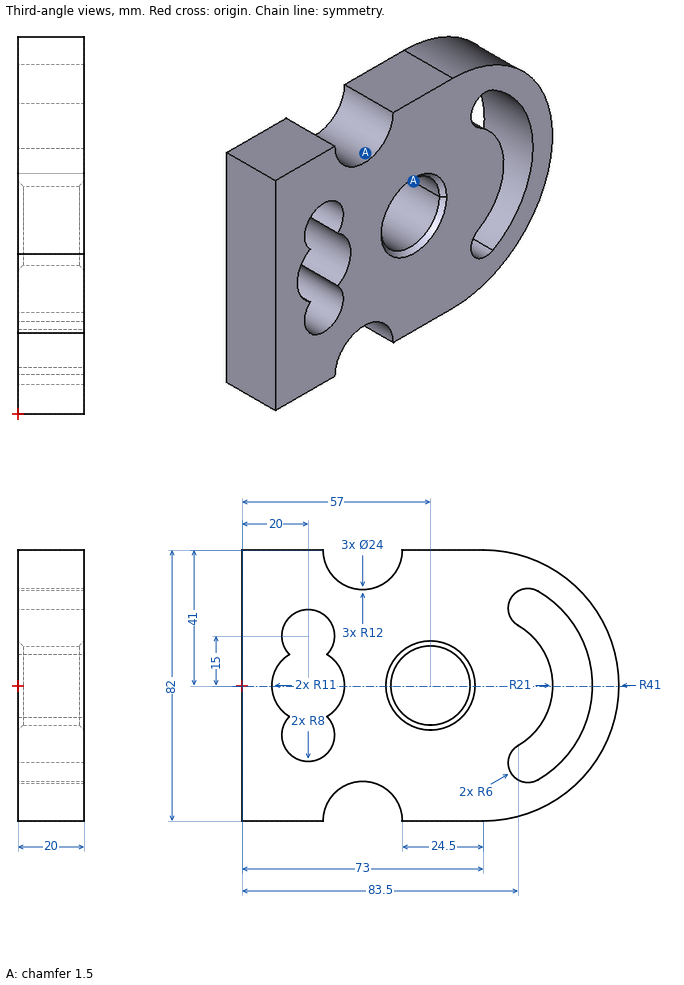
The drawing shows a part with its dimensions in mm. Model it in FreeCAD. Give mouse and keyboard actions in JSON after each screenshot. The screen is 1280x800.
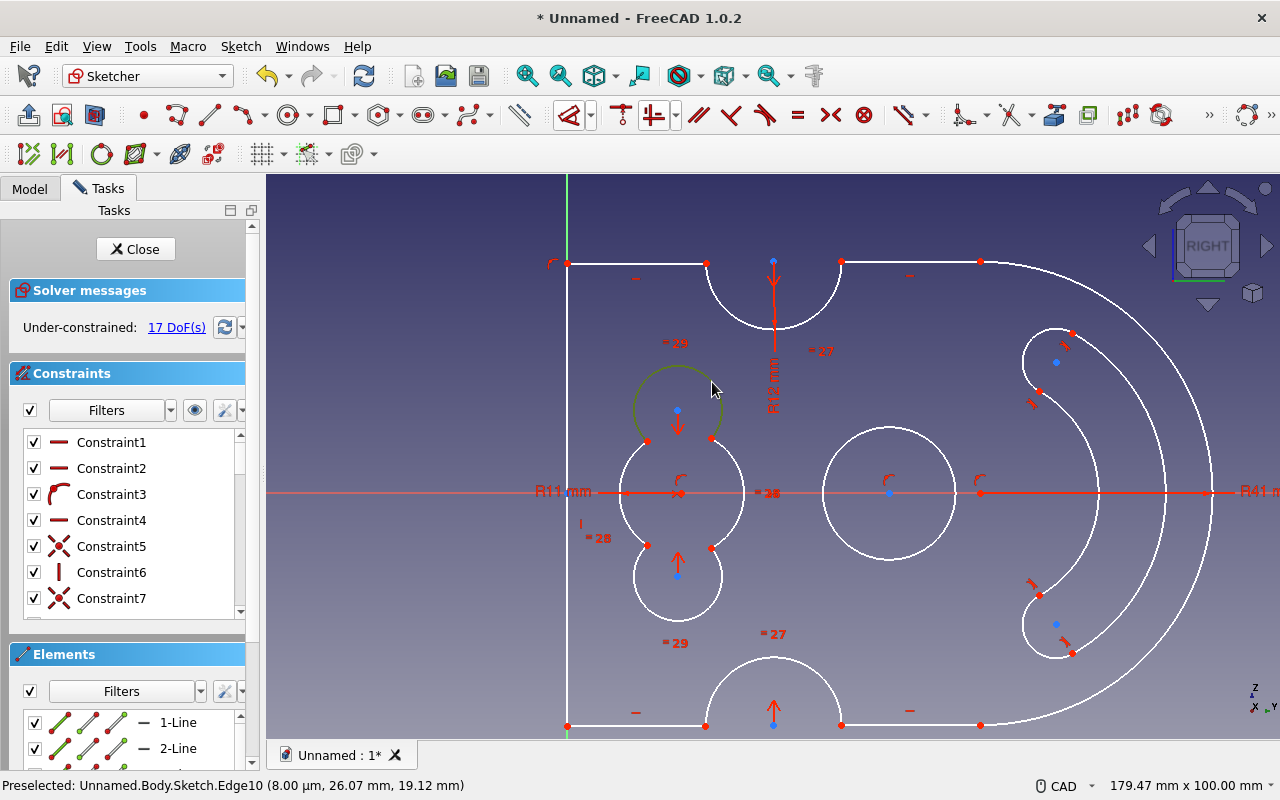
{"action": "key", "text": "k r"}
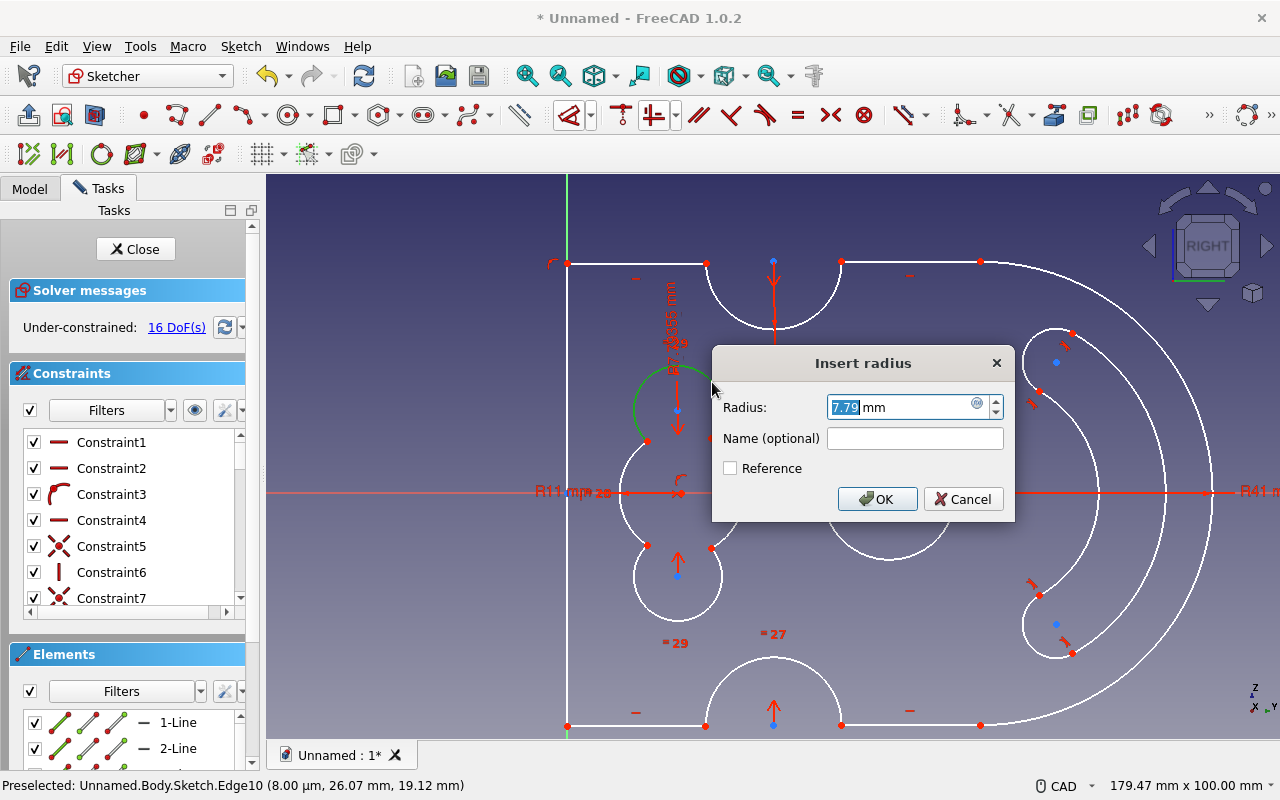
{"action": "type", "text": "8"}
{"action": "key", "text": "Return"}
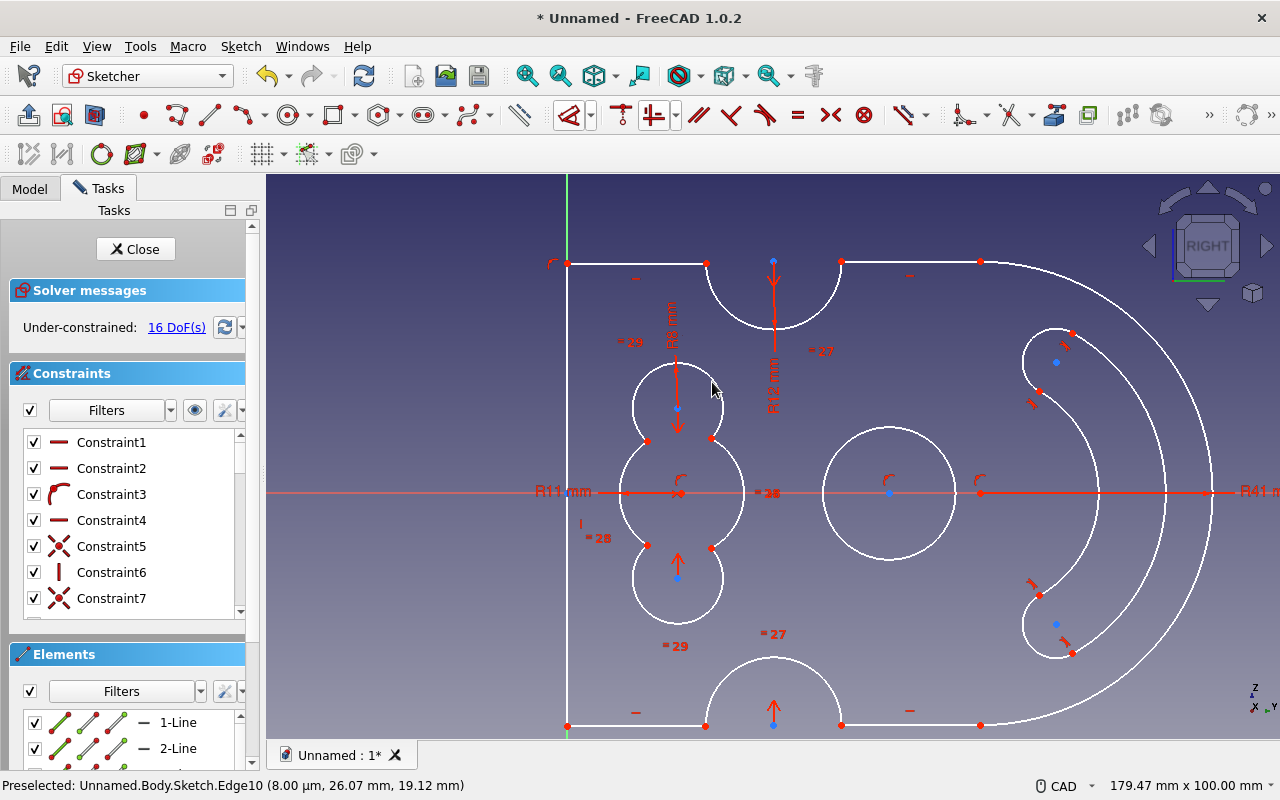
{"action": "left_click", "coordinate": [1088, 541]}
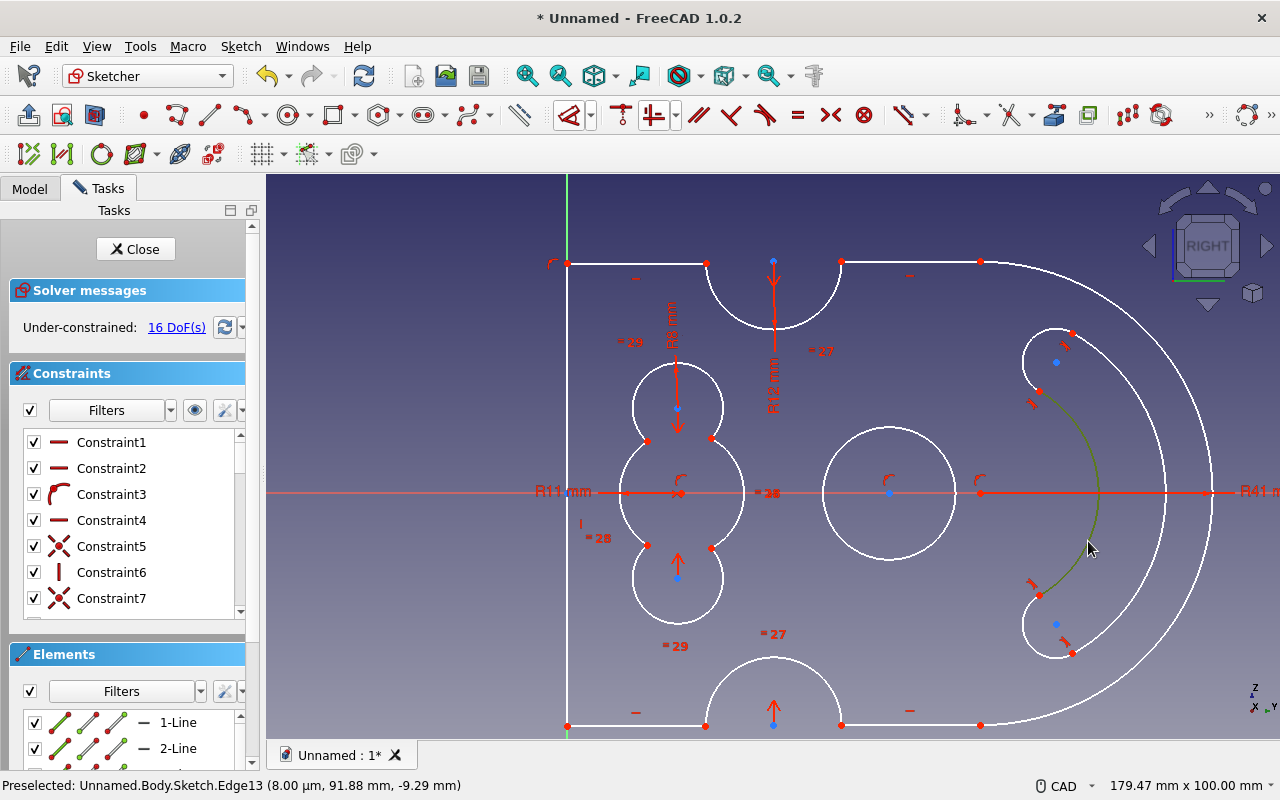
{"action": "key", "text": "k r"}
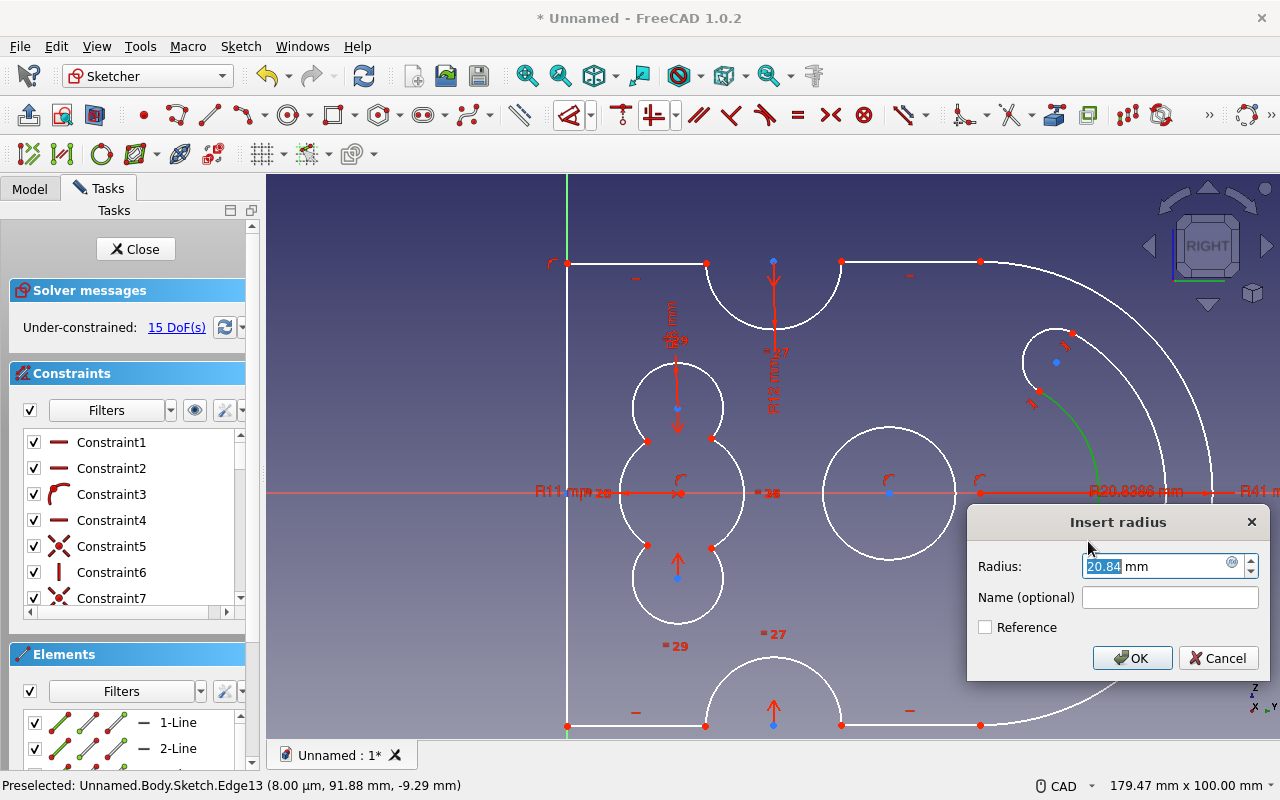
{"action": "type", "text": "21"}
{"action": "key", "text": "Return"}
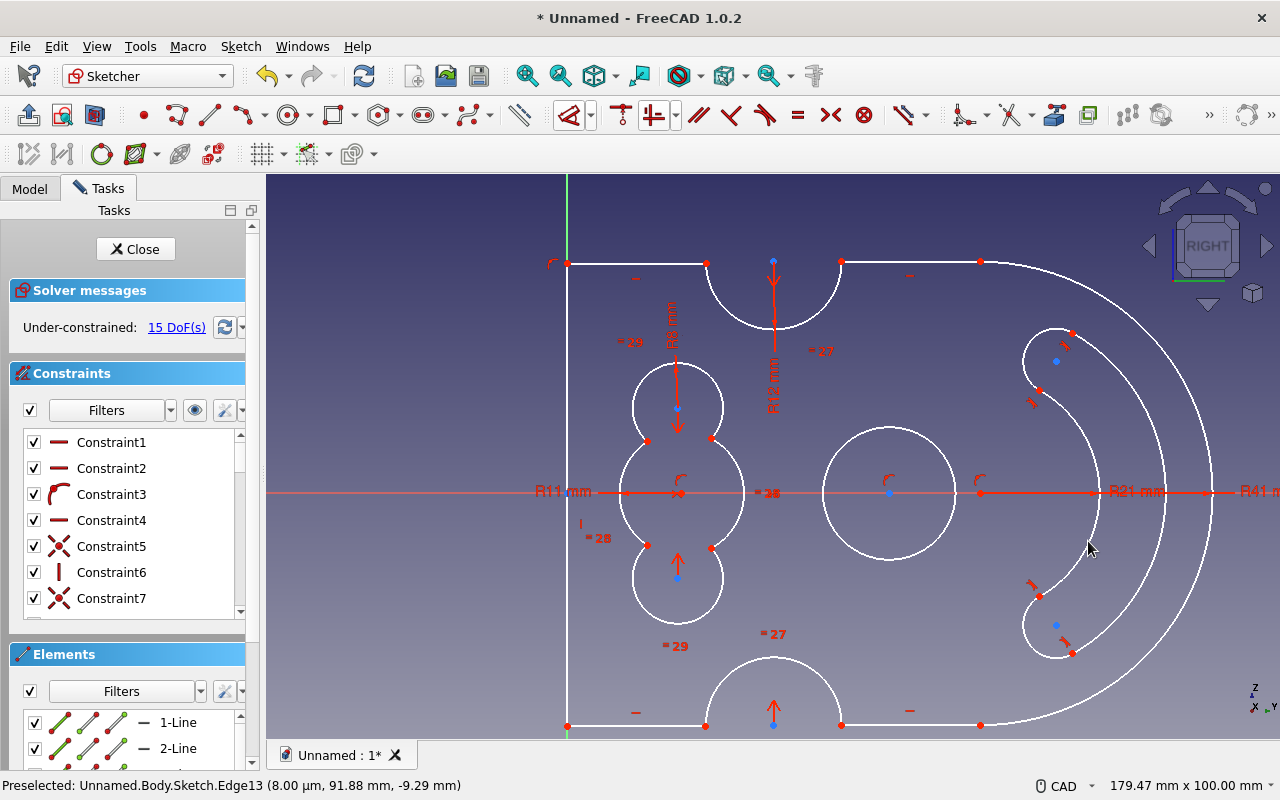
{"action": "left_click", "coordinate": [1043, 332]}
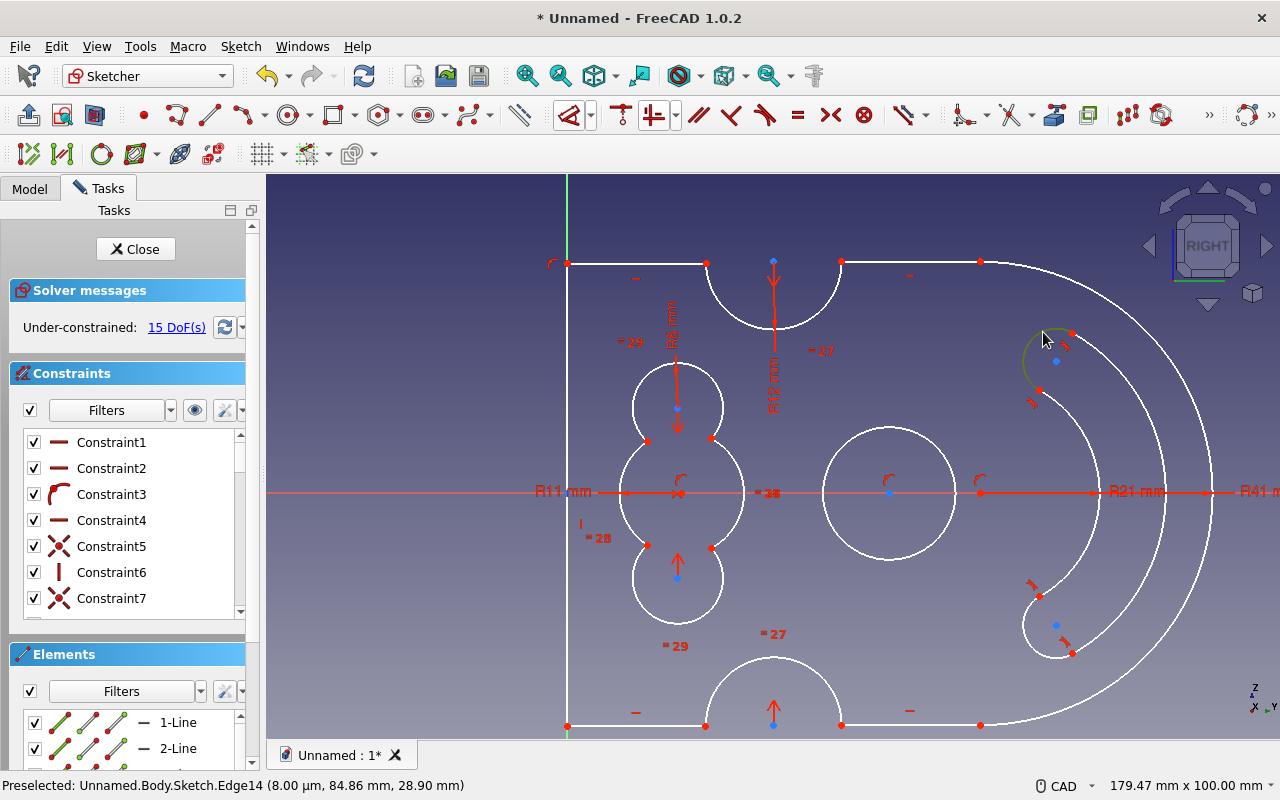
{"action": "key", "text": "k r"}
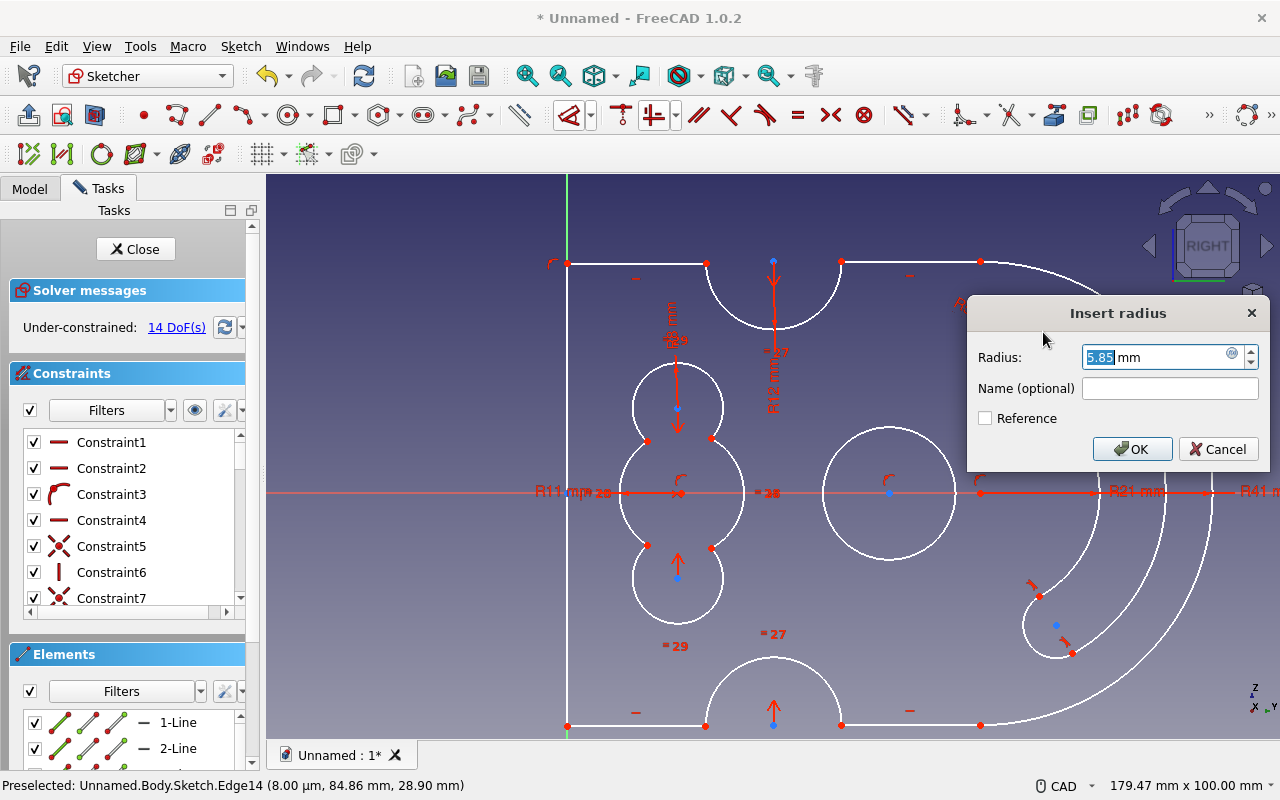
{"action": "type", "text": "6"}
{"action": "key", "text": "Return"}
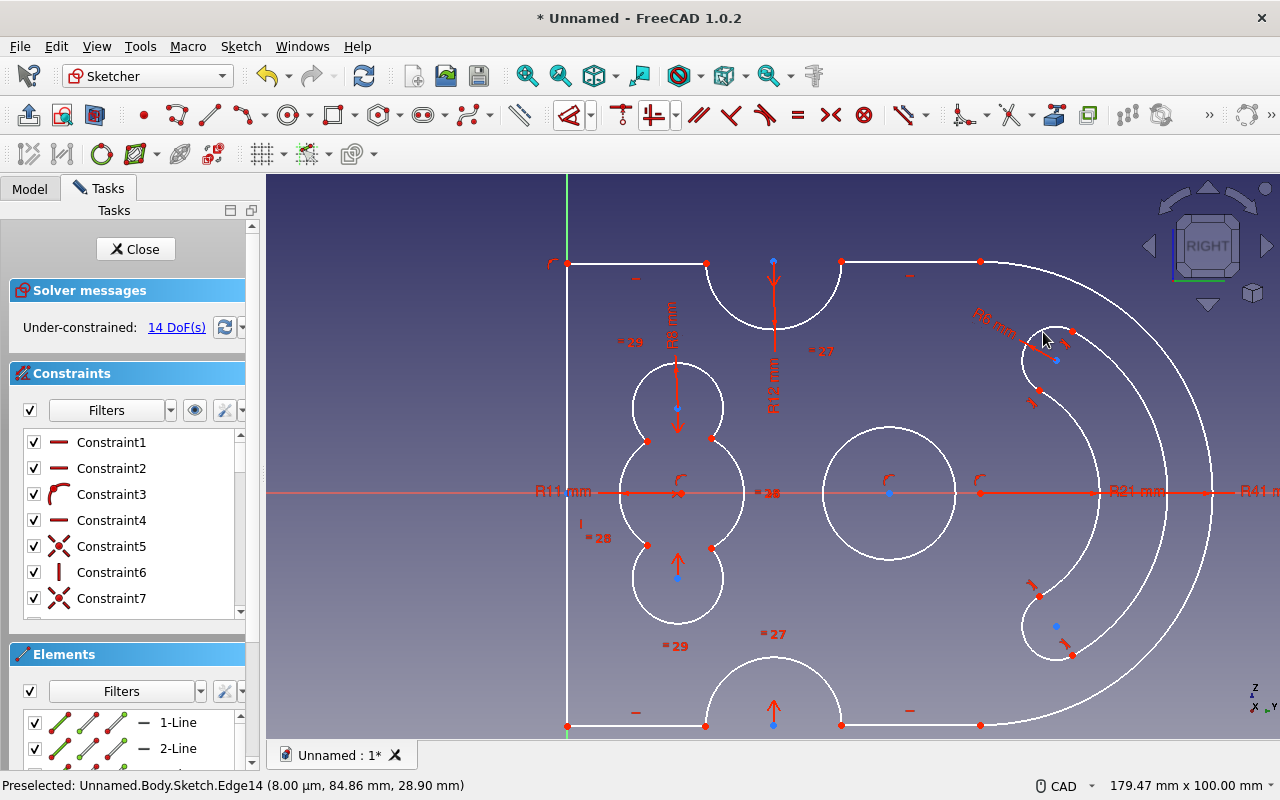
{"action": "left_click", "coordinate": [936, 446]}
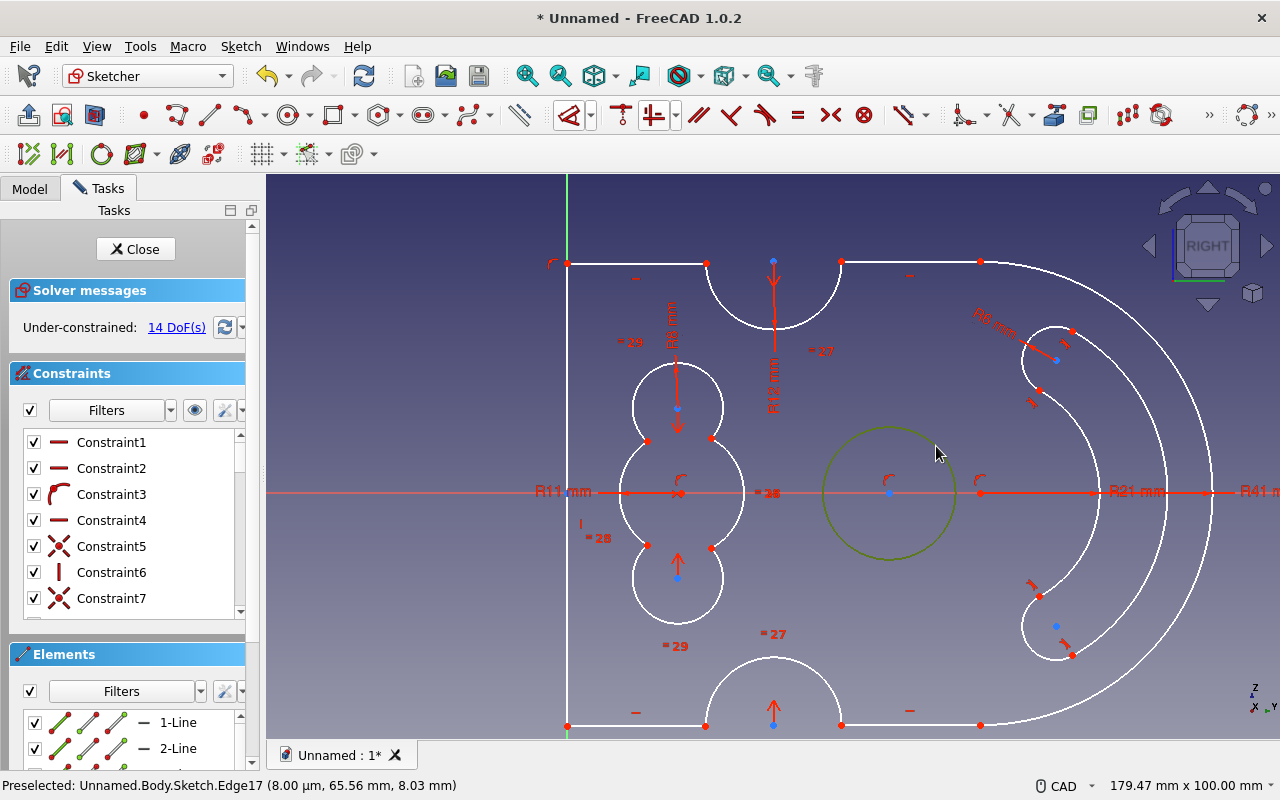
{"action": "key", "text": "k o"}